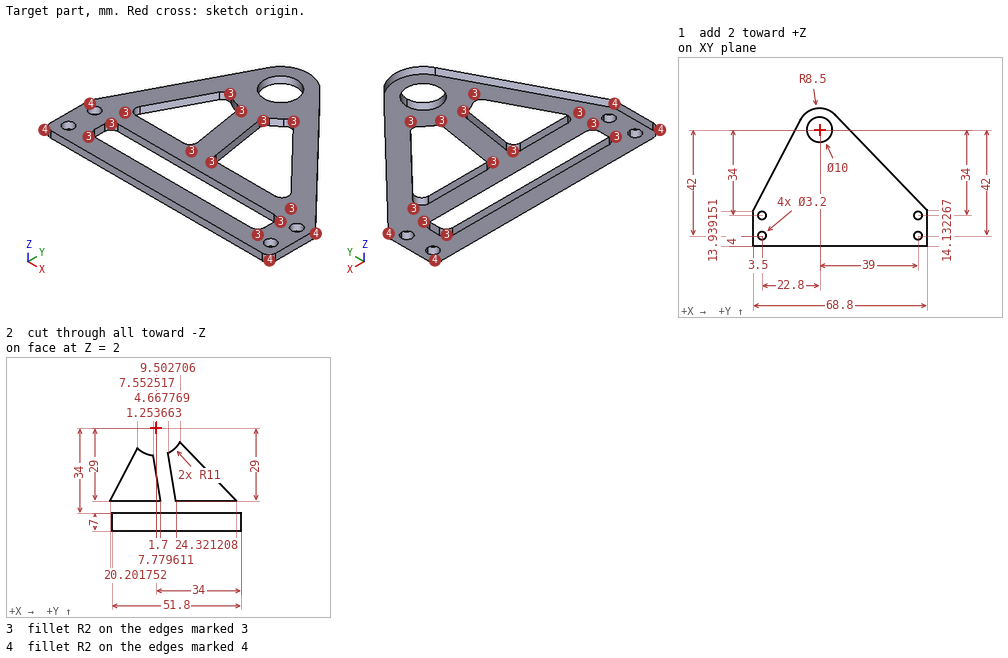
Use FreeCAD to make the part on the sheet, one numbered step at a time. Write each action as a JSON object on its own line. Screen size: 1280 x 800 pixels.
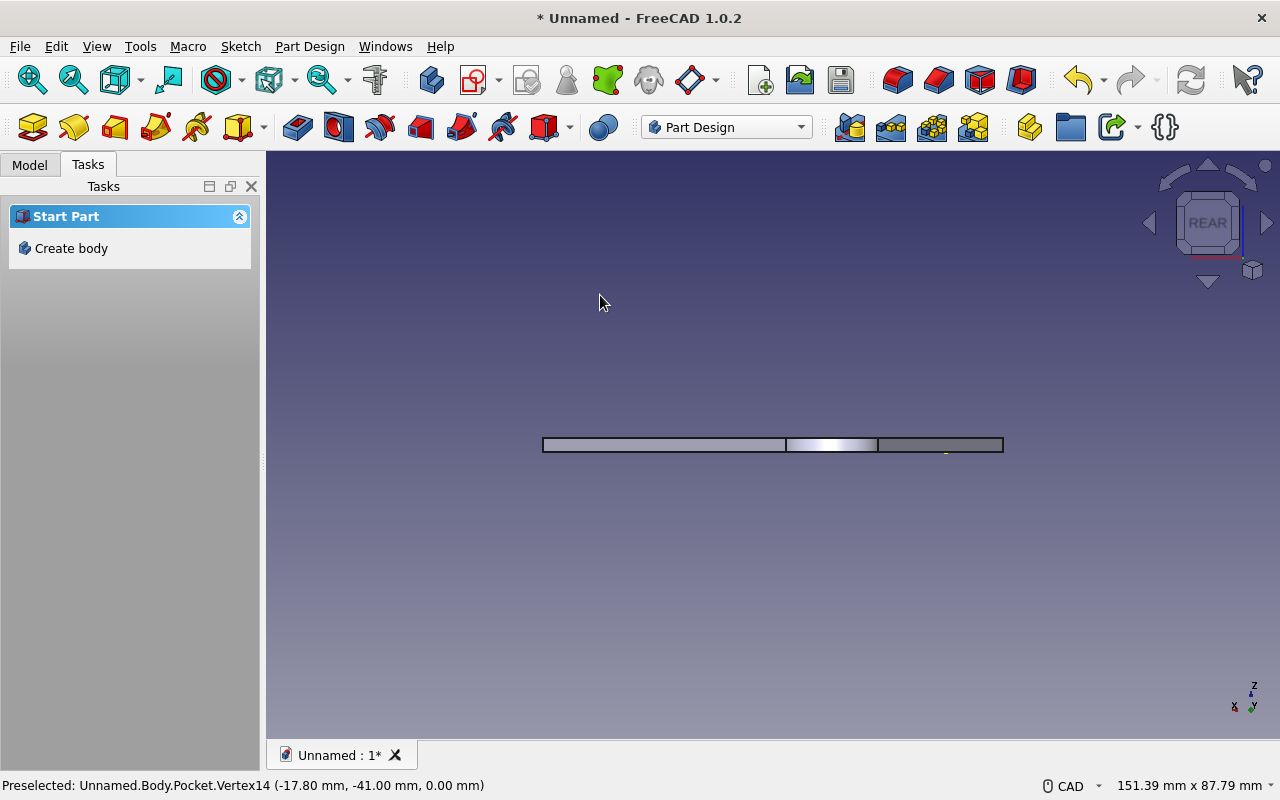
{"action": "scroll", "coordinate": [946, 444], "scroll_direction": "up", "scroll_amount": 6}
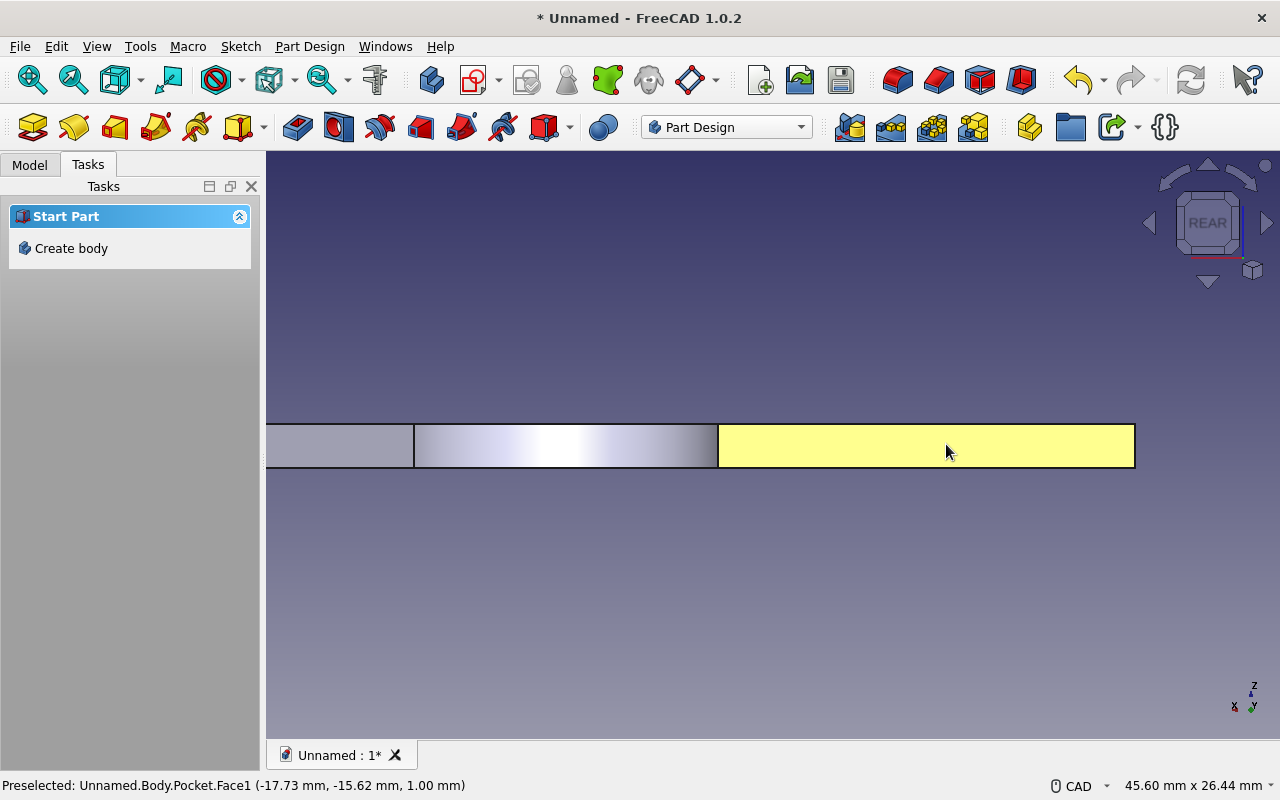
{"action": "left_click", "coordinate": [33, 80]}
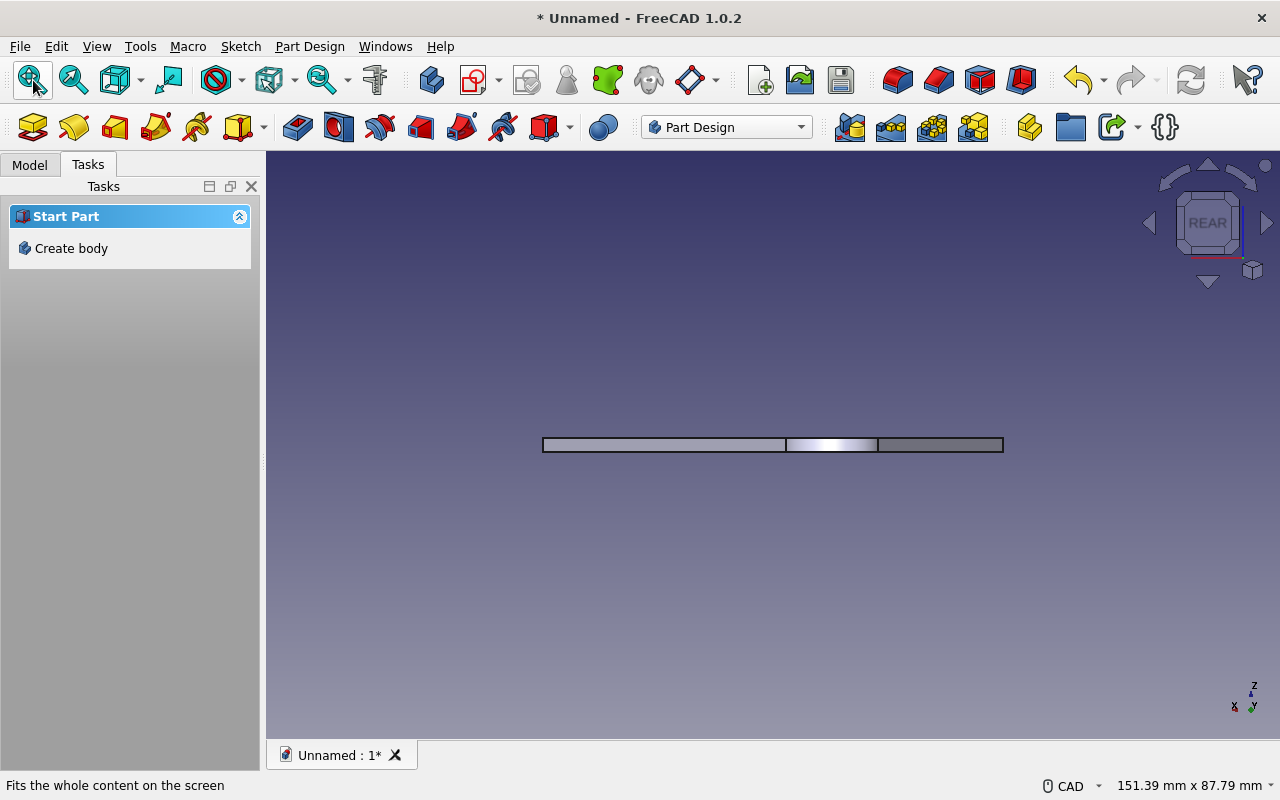
{"action": "key", "text": "6"}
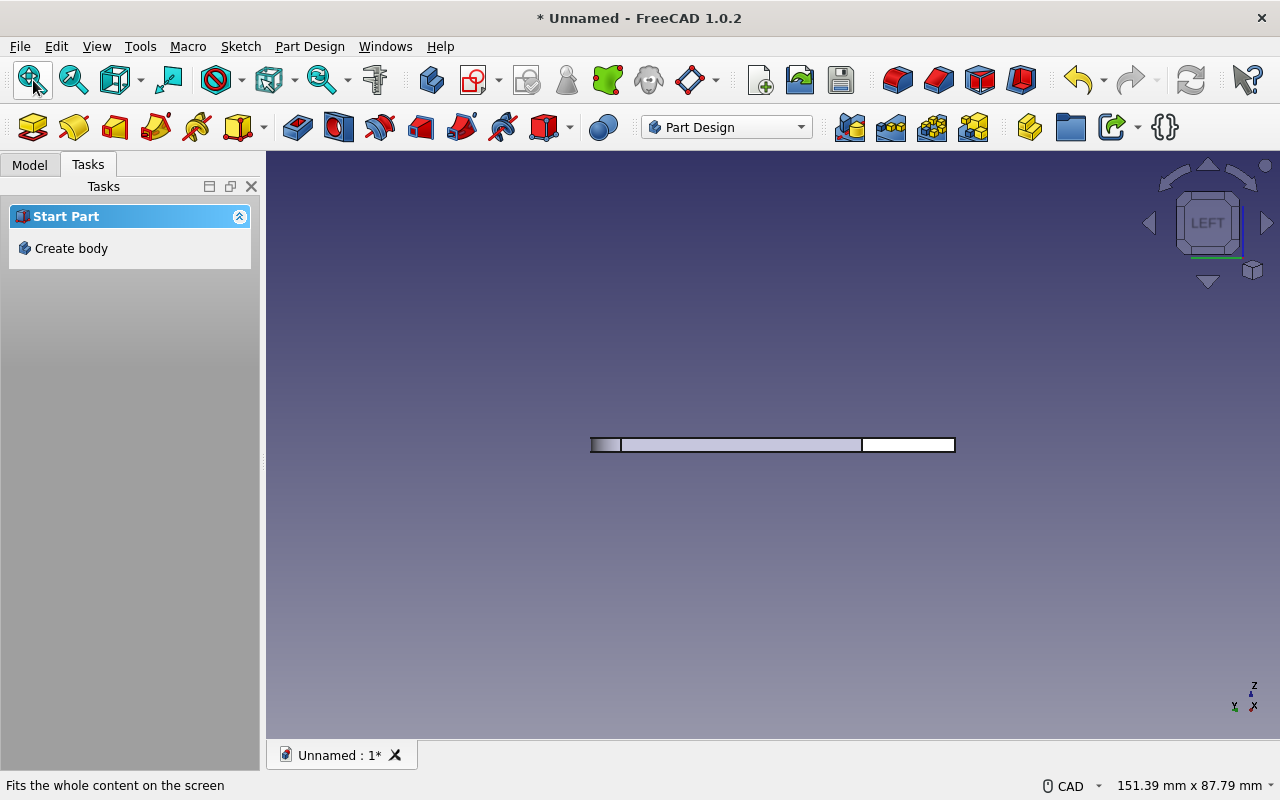
{"action": "left_click", "coordinate": [33, 80]}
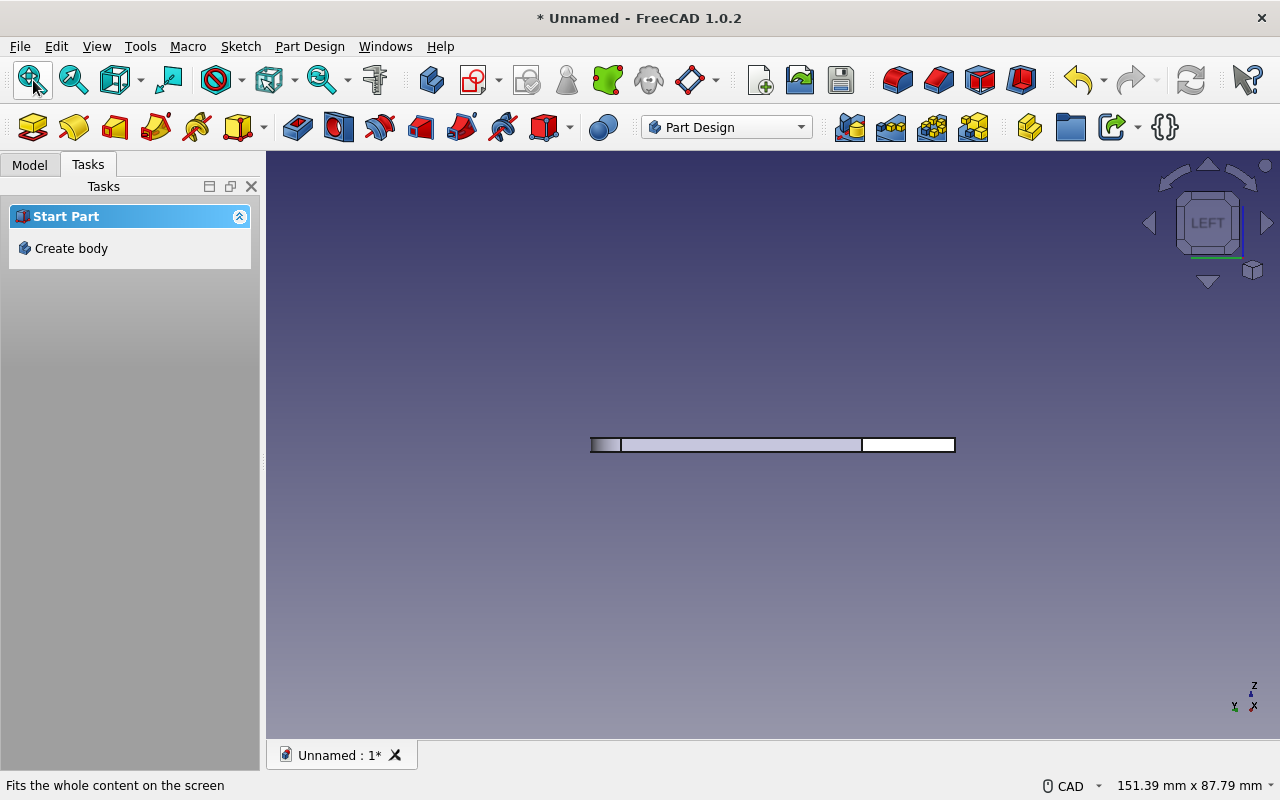
{"action": "scroll", "coordinate": [922, 444], "scroll_direction": "up", "scroll_amount": 6}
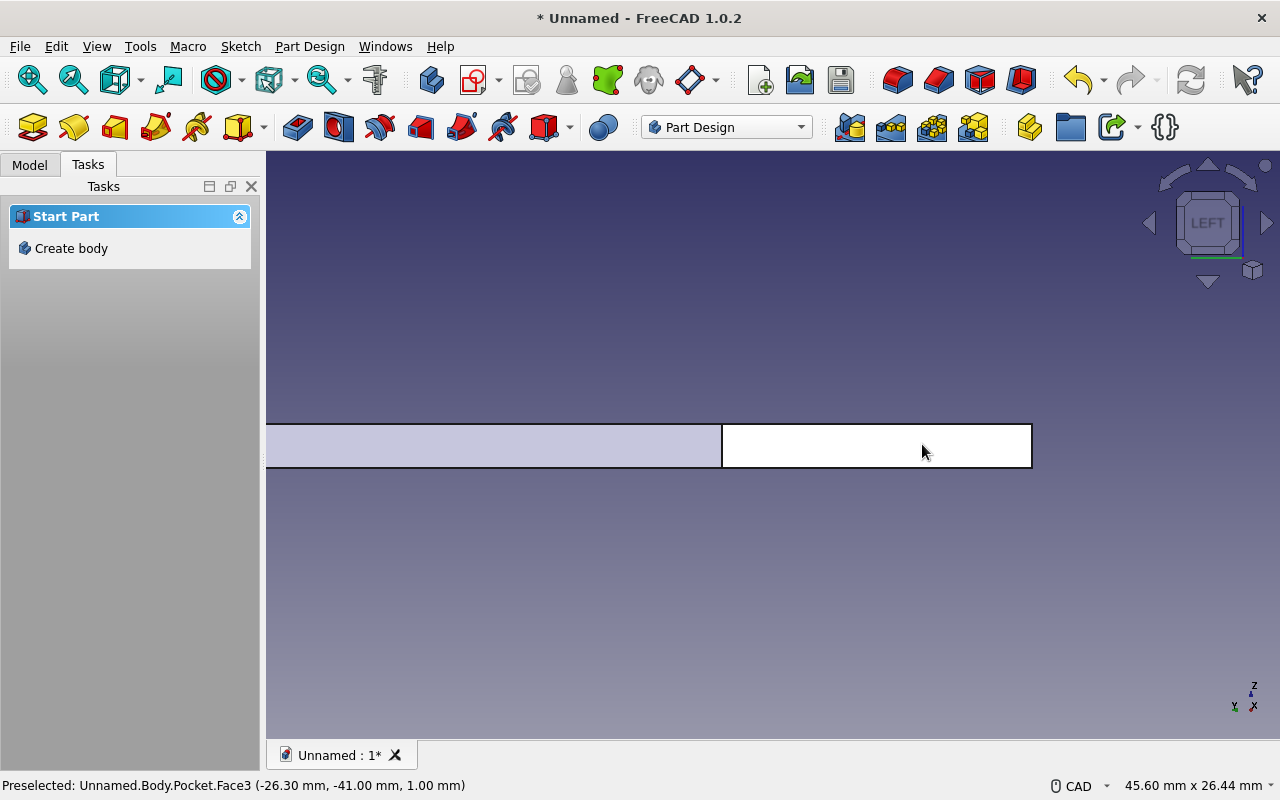
{"action": "left_click", "coordinate": [33, 80]}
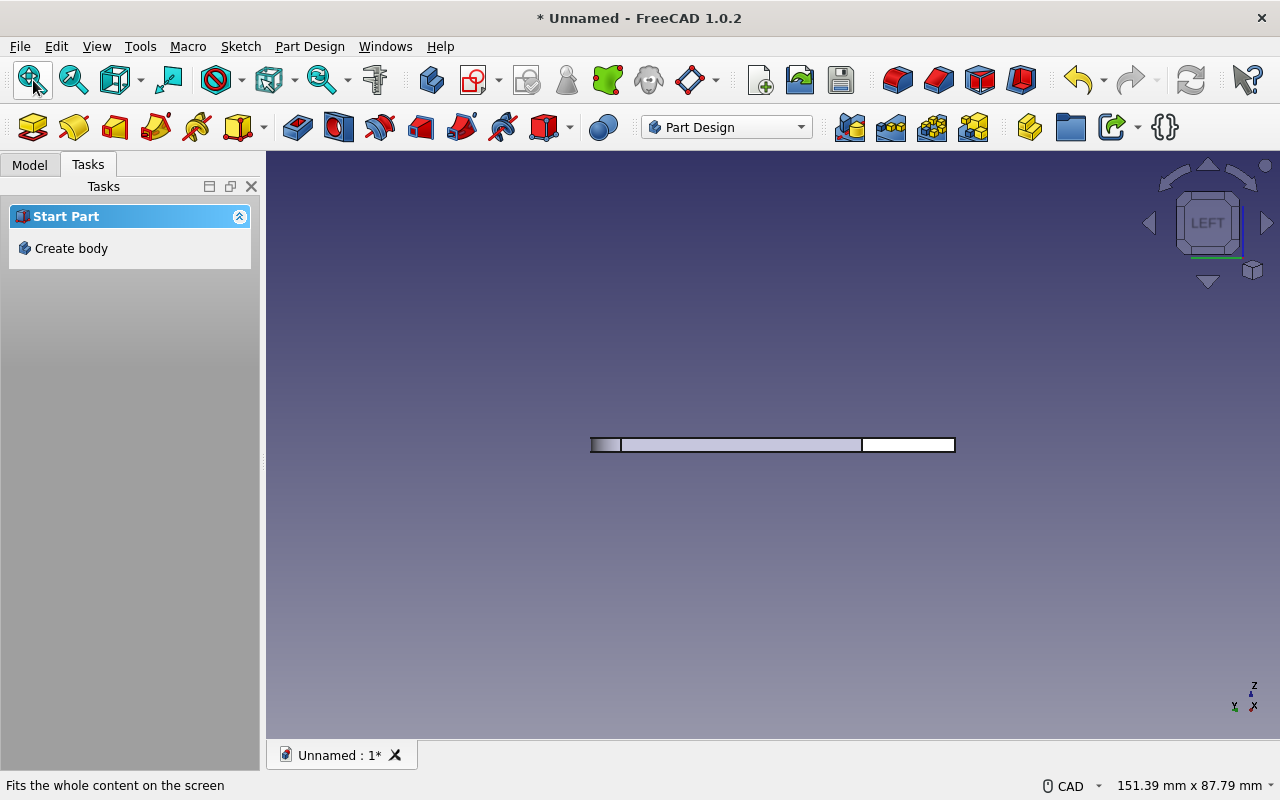
{"action": "key", "text": "v 3"}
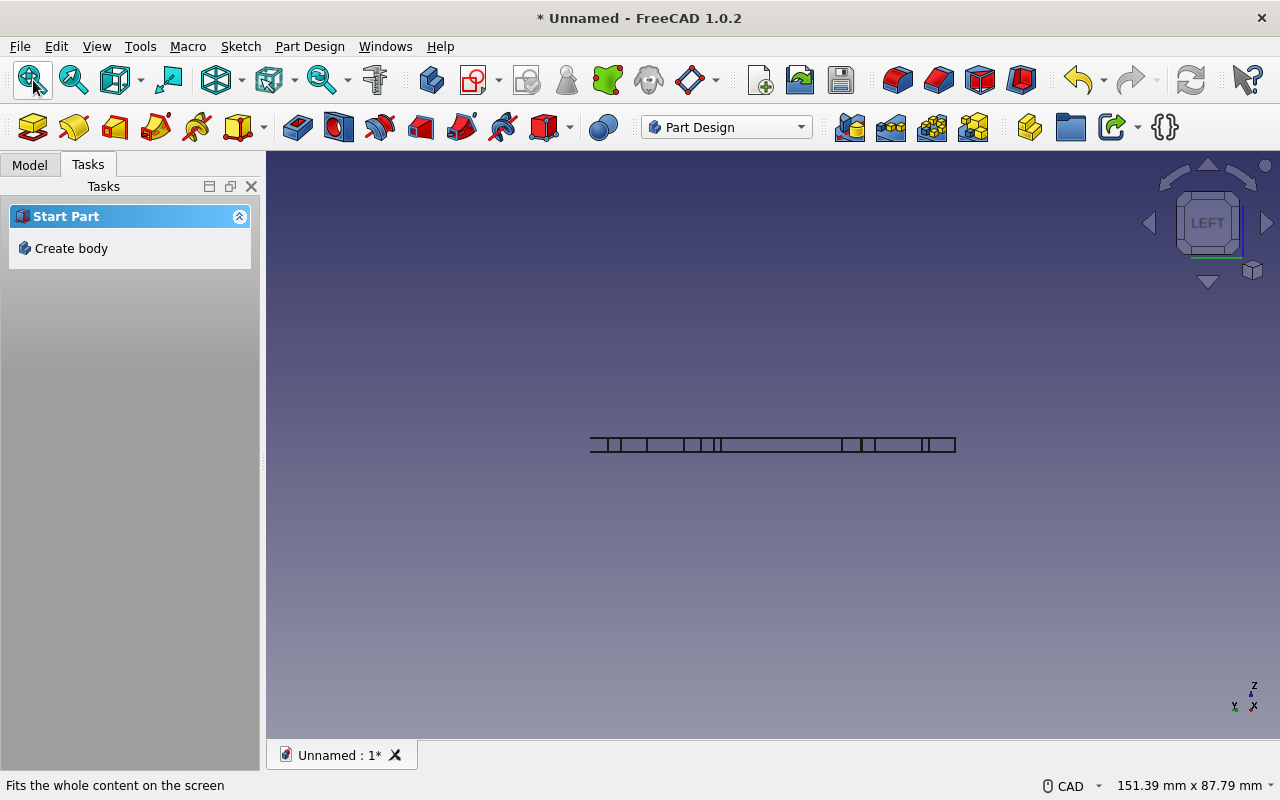
{"action": "key", "text": "0"}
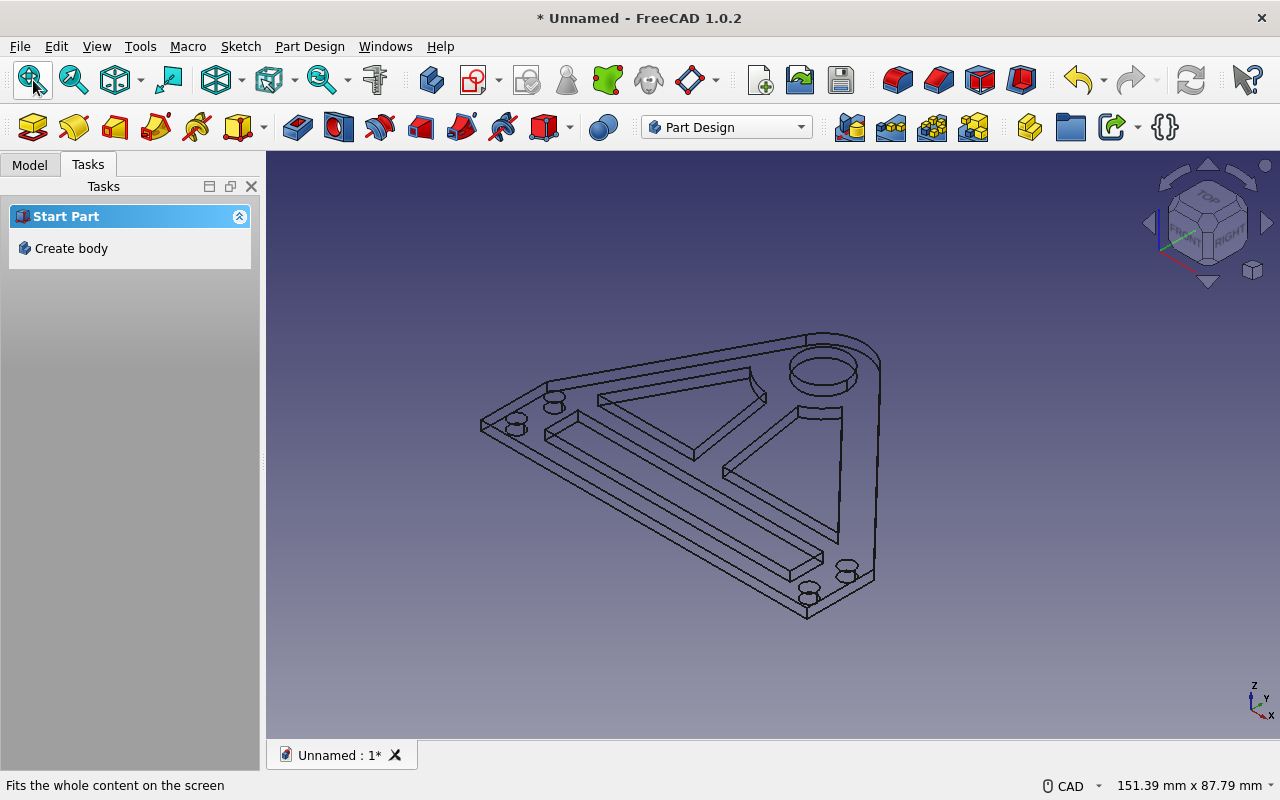
{"action": "left_click", "coordinate": [545, 436]}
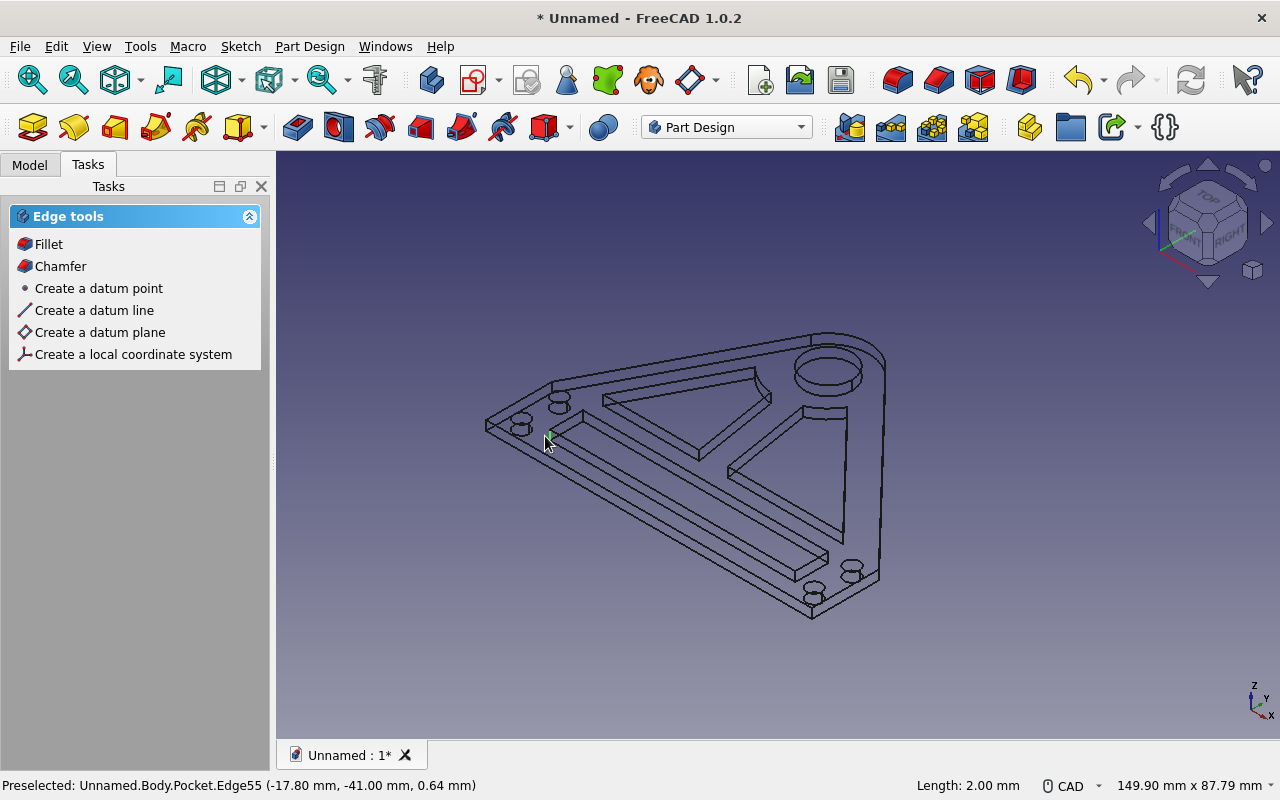
{"action": "left_click", "coordinate": [583, 417], "text": "ctrl"}